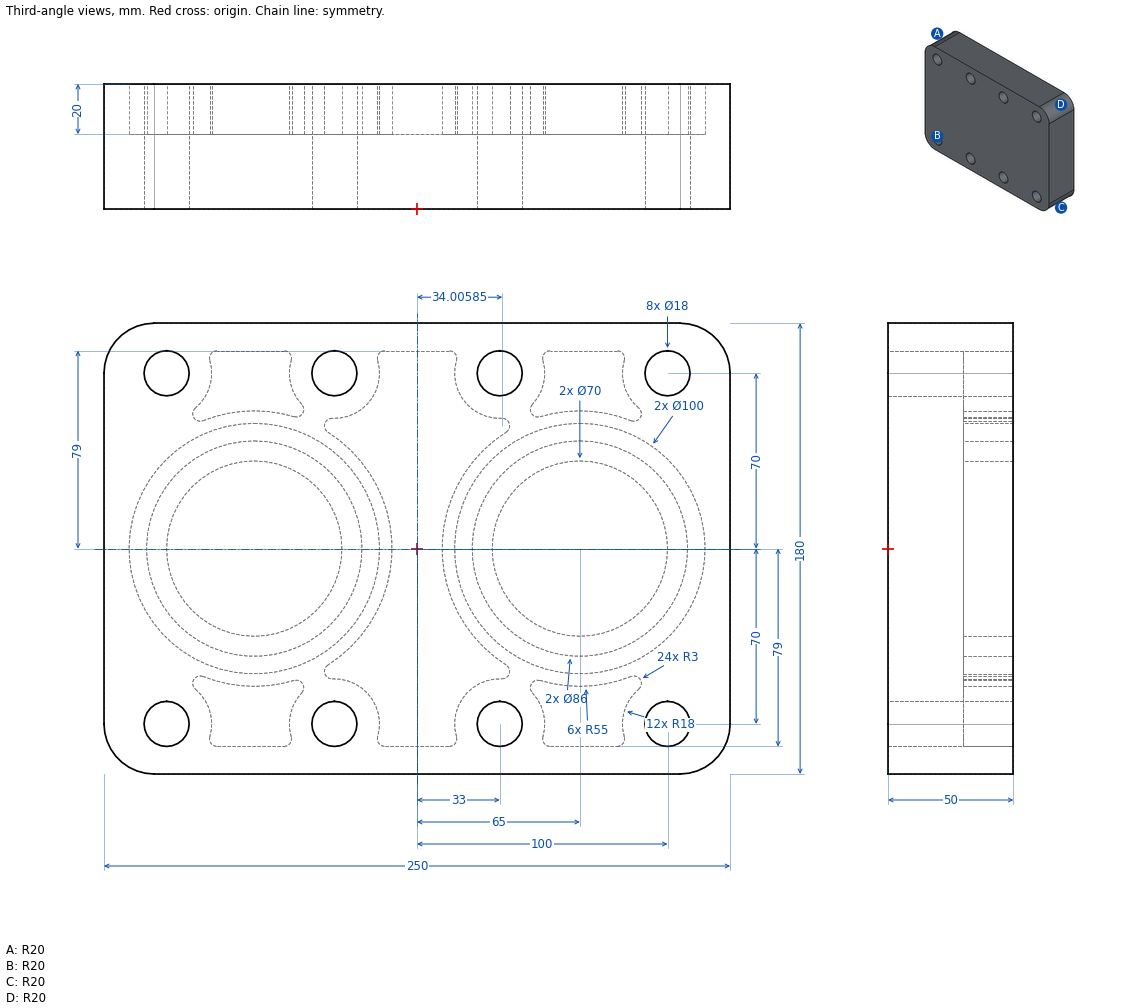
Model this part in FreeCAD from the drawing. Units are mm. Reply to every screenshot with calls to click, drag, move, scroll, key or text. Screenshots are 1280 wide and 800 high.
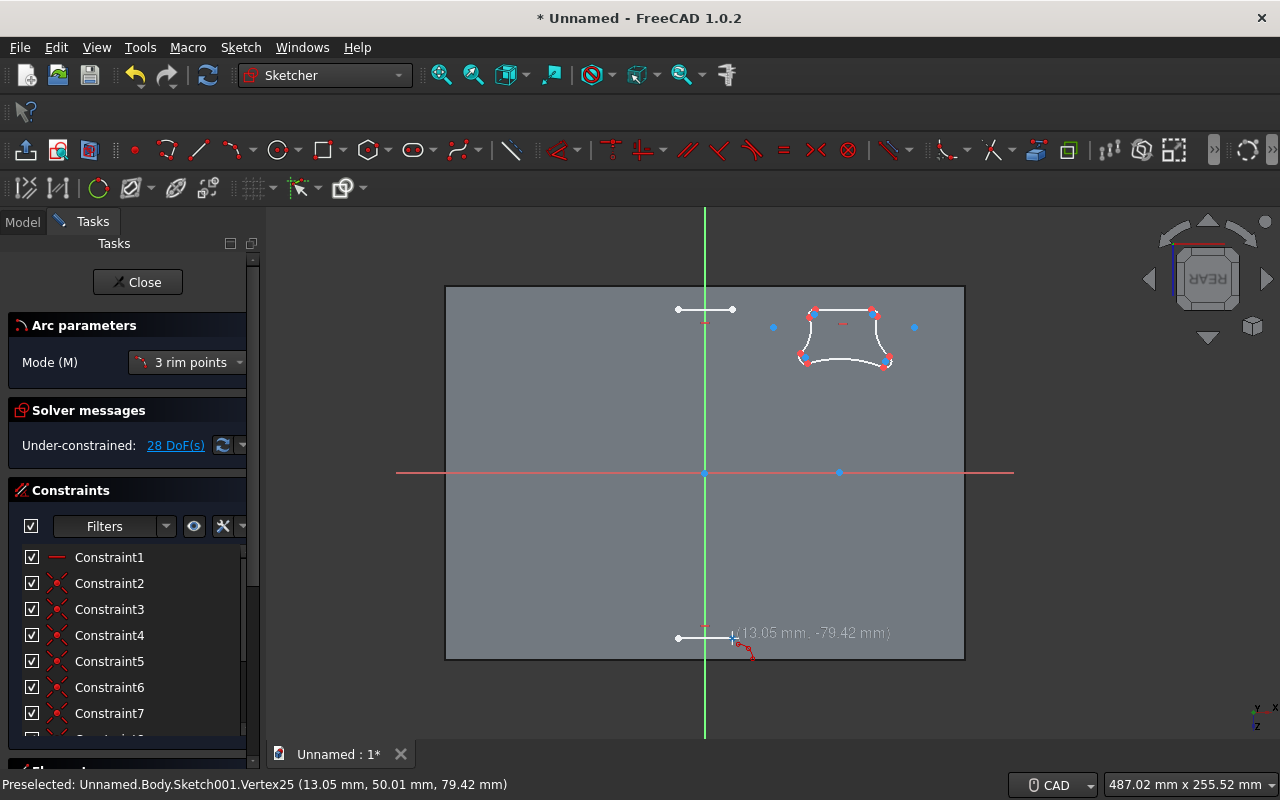
scroll(738, 629, up, 3)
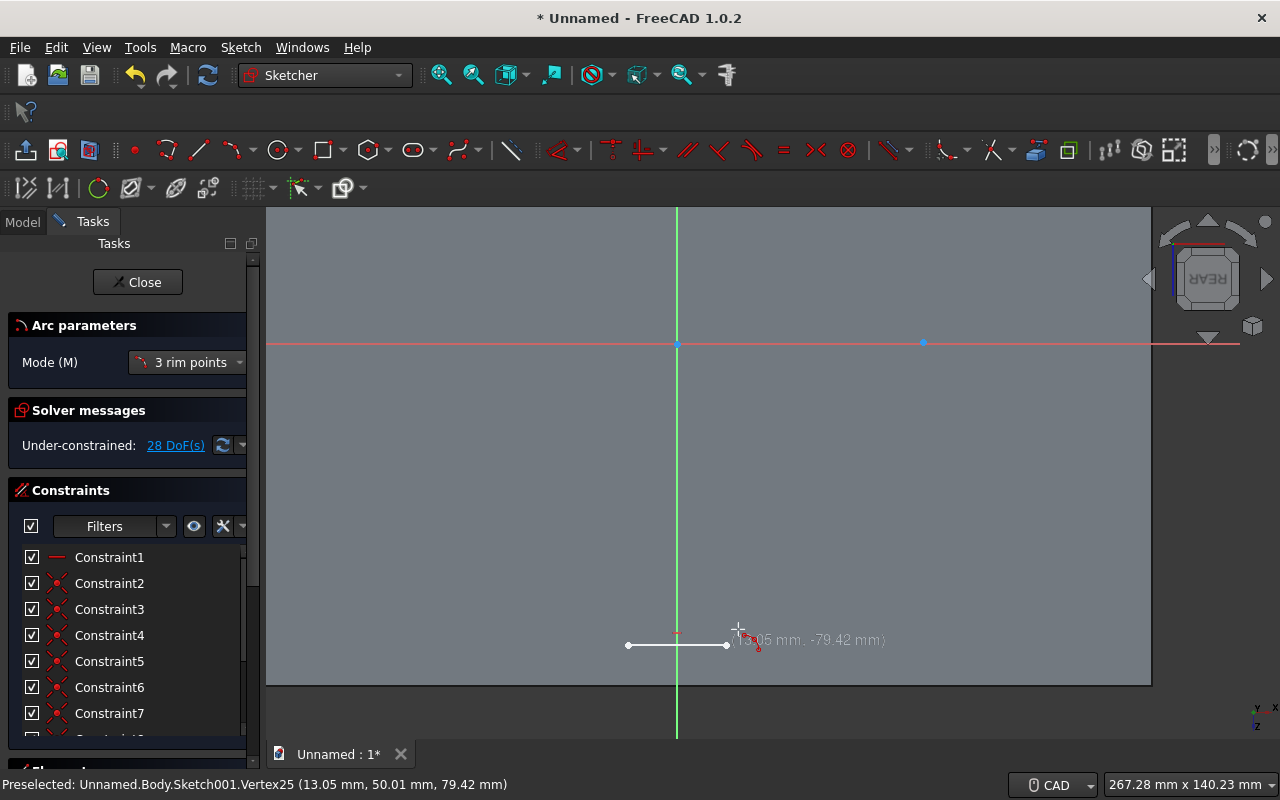
click(737, 629)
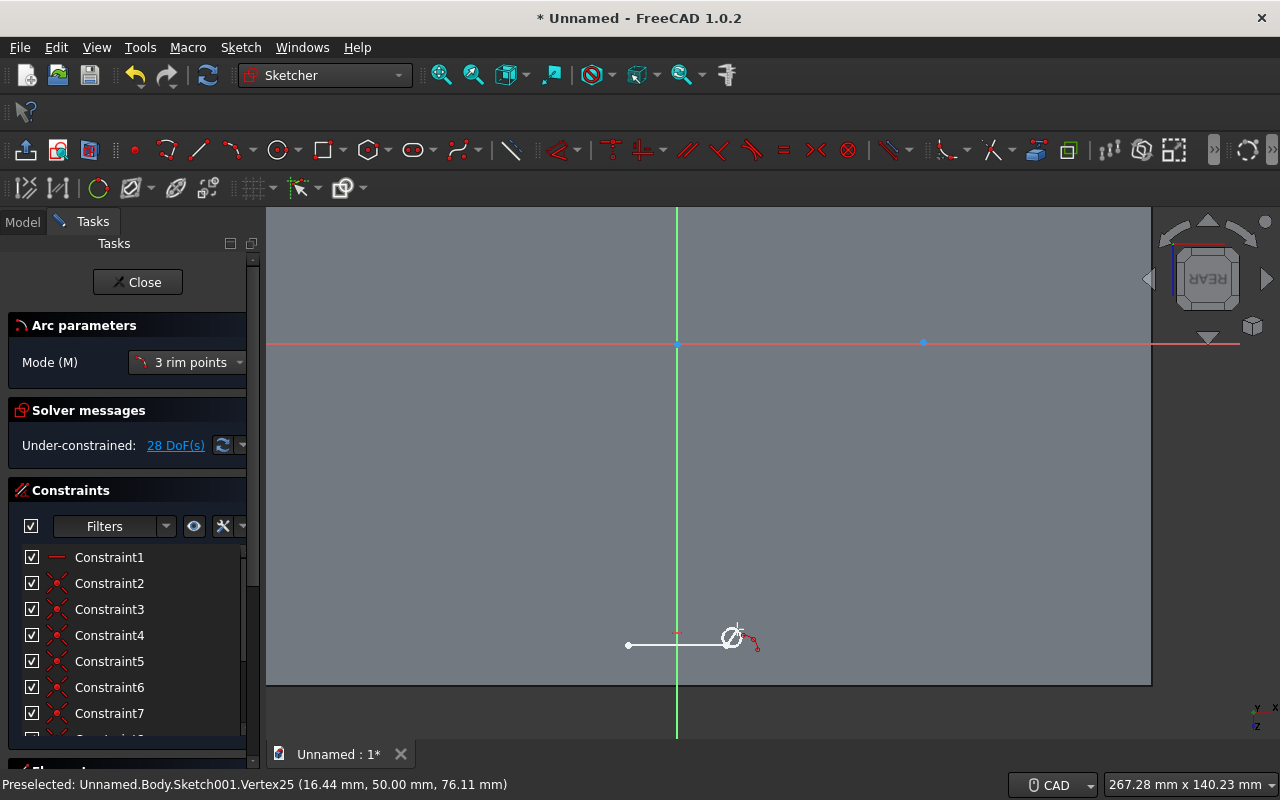
scroll(735, 639, up, 7)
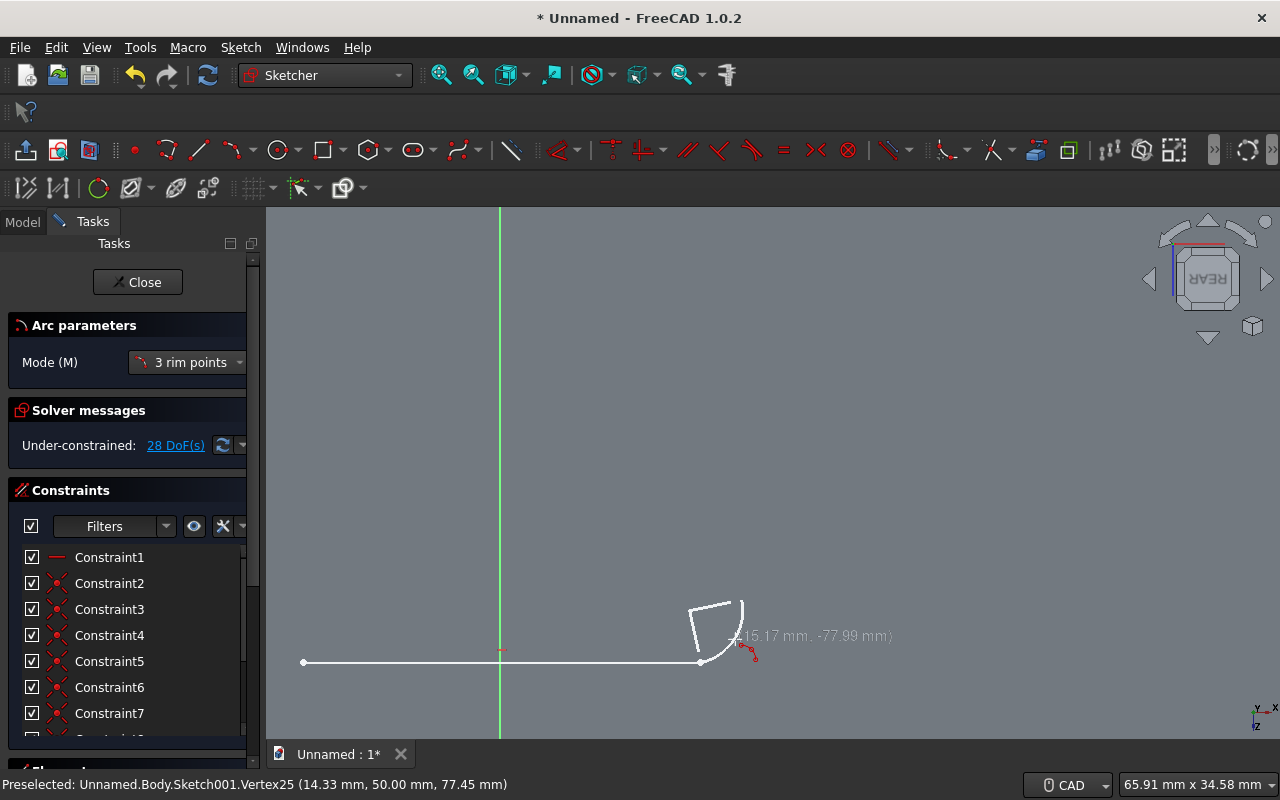
click(735, 638)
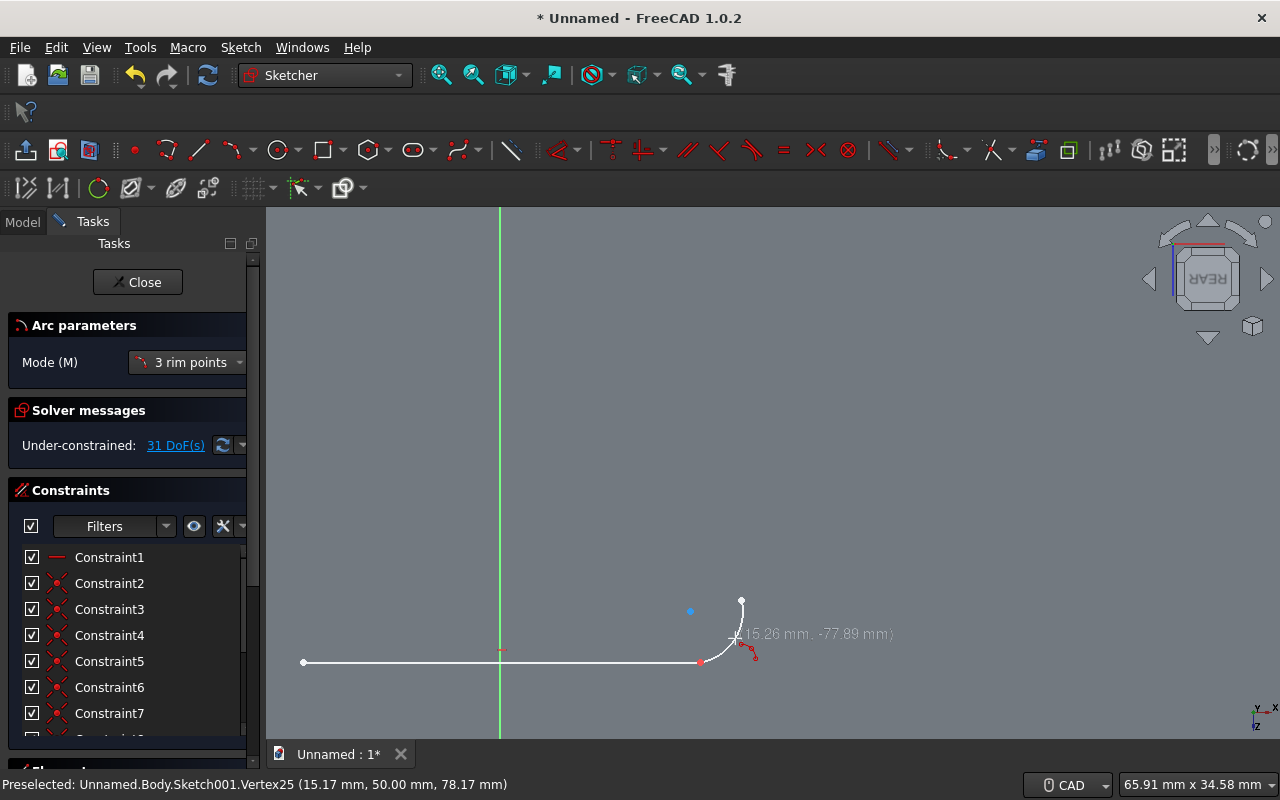
scroll(736, 635, down, 10)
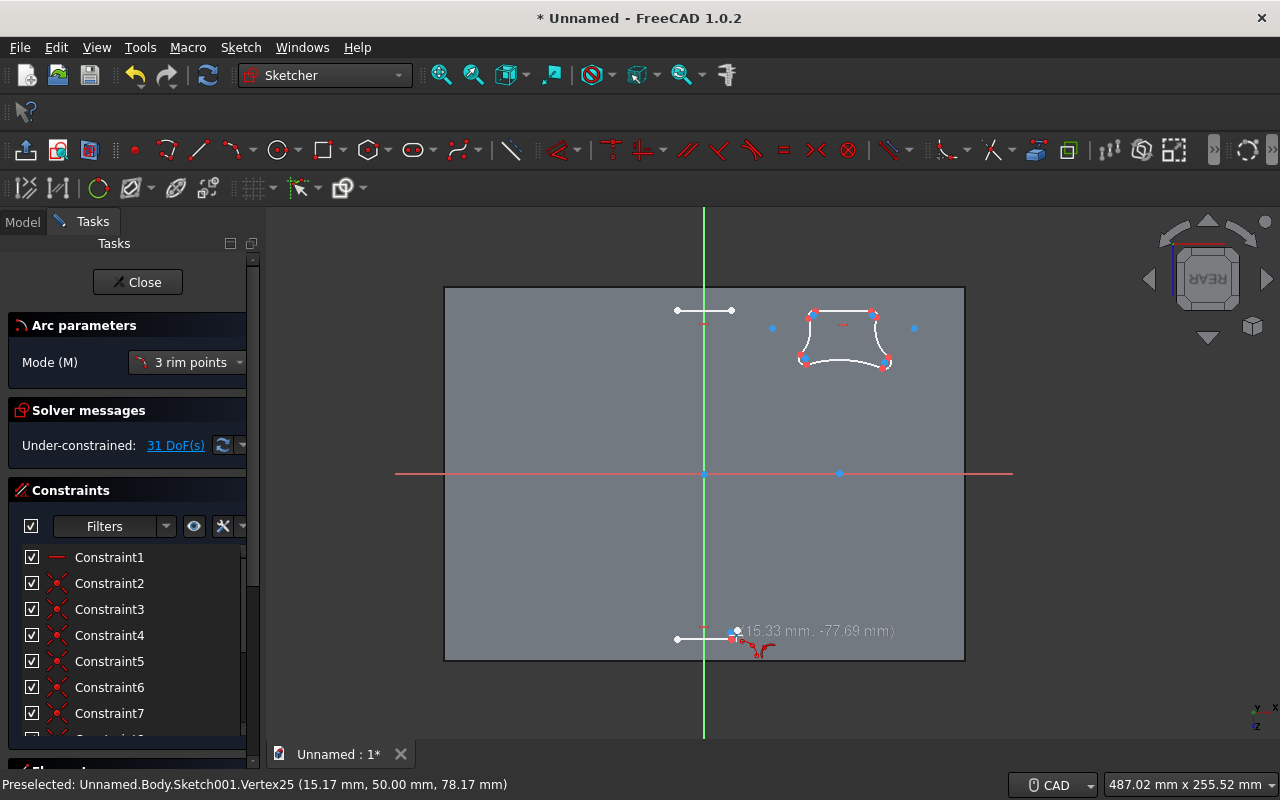
scroll(737, 631, up, 5)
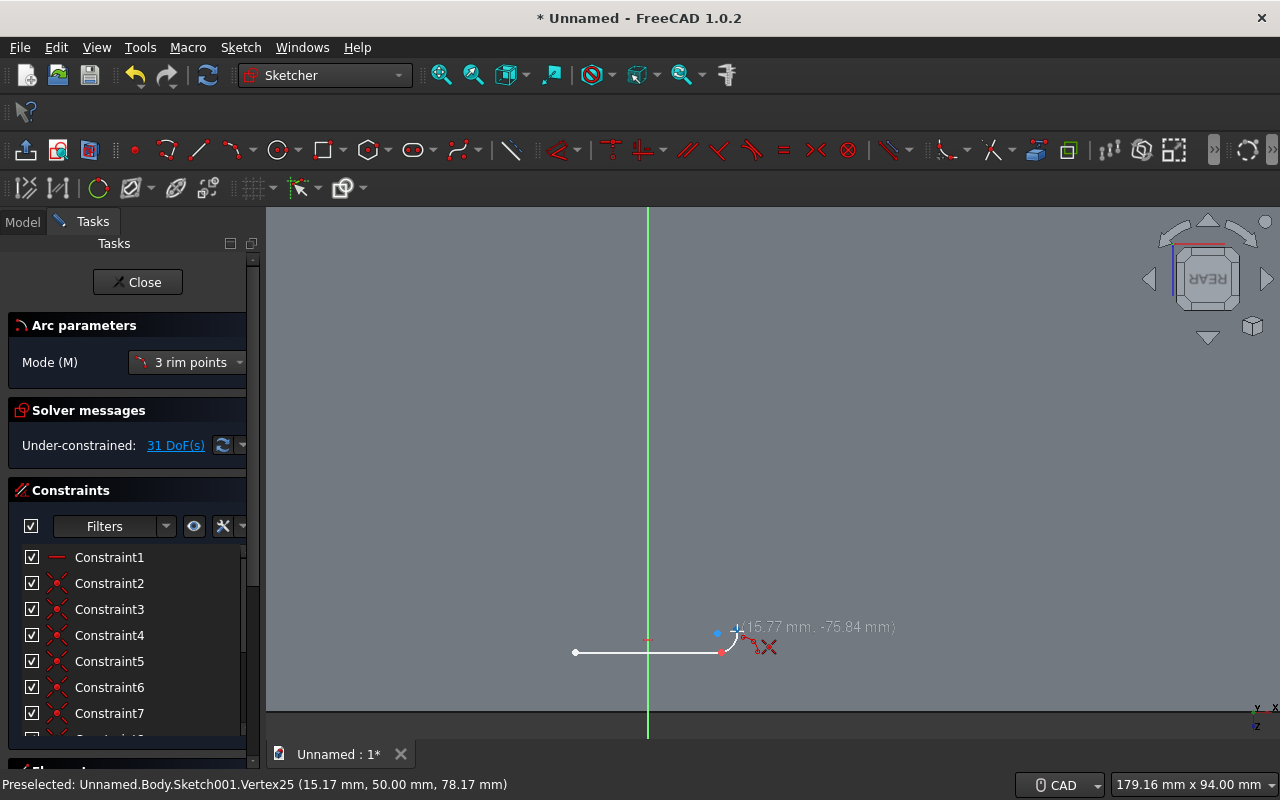
click(737, 630)
click(839, 497)
click(754, 536)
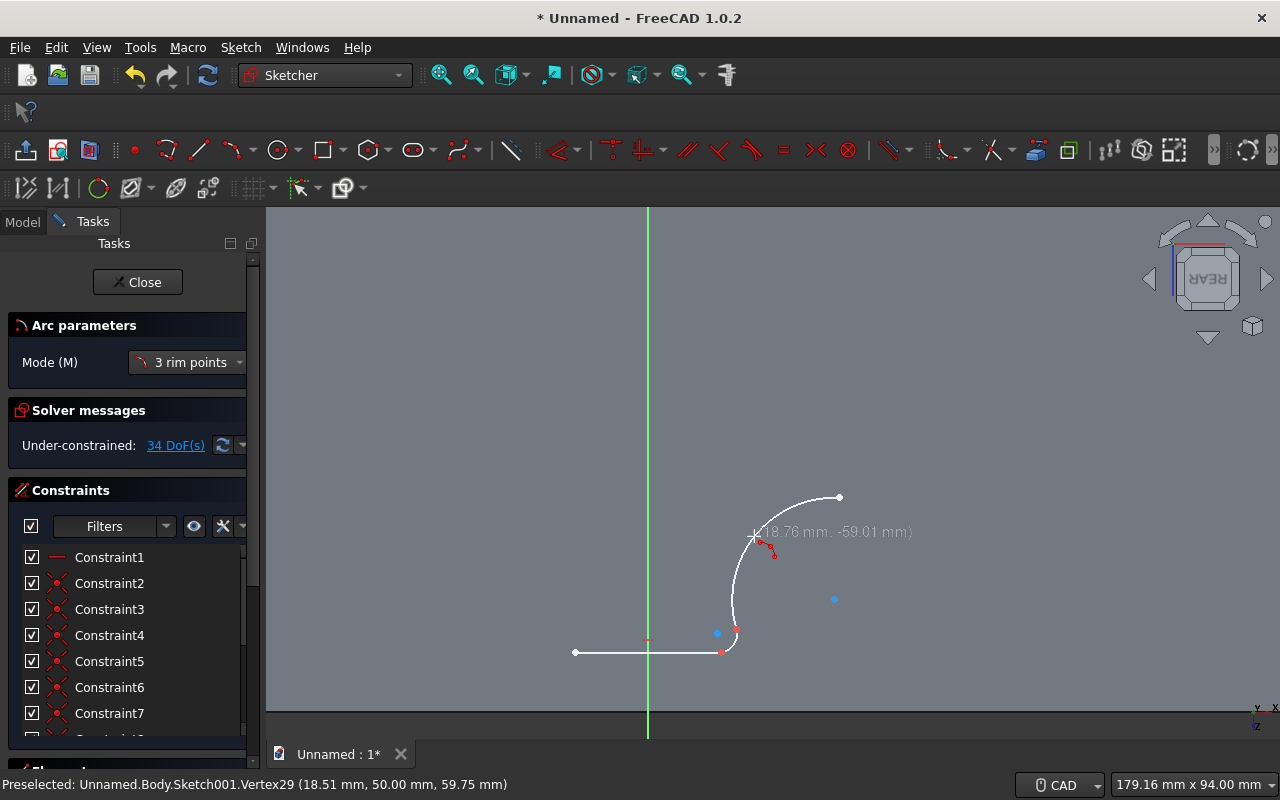
click(839, 498)
click(849, 466)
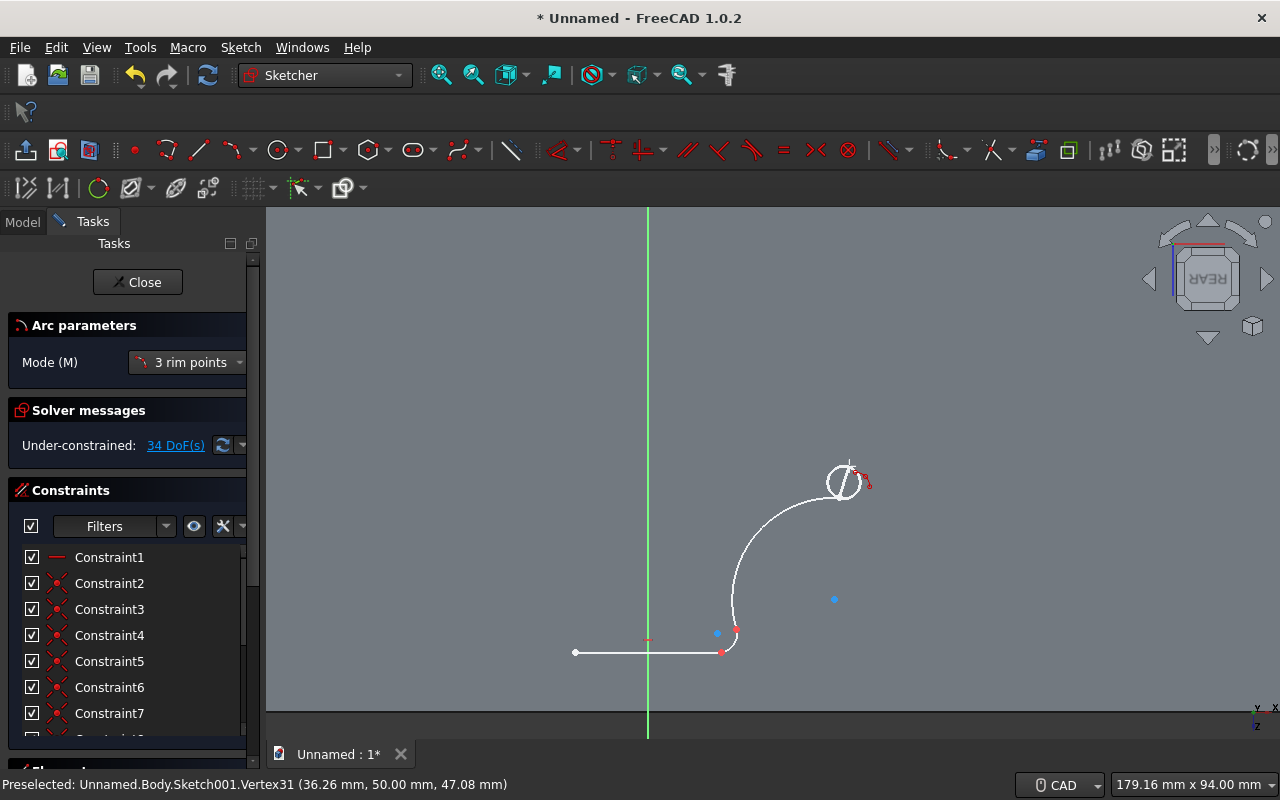
scroll(856, 486, up, 2)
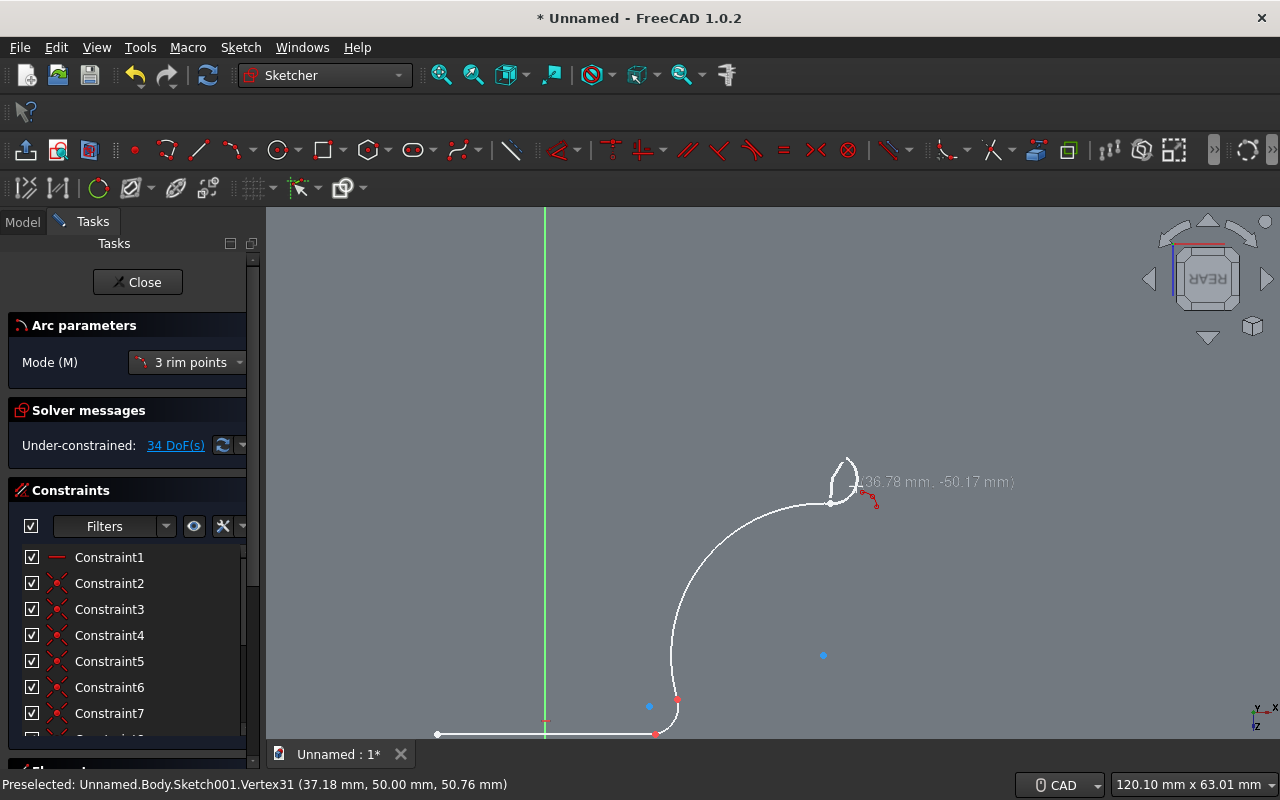
click(856, 485)